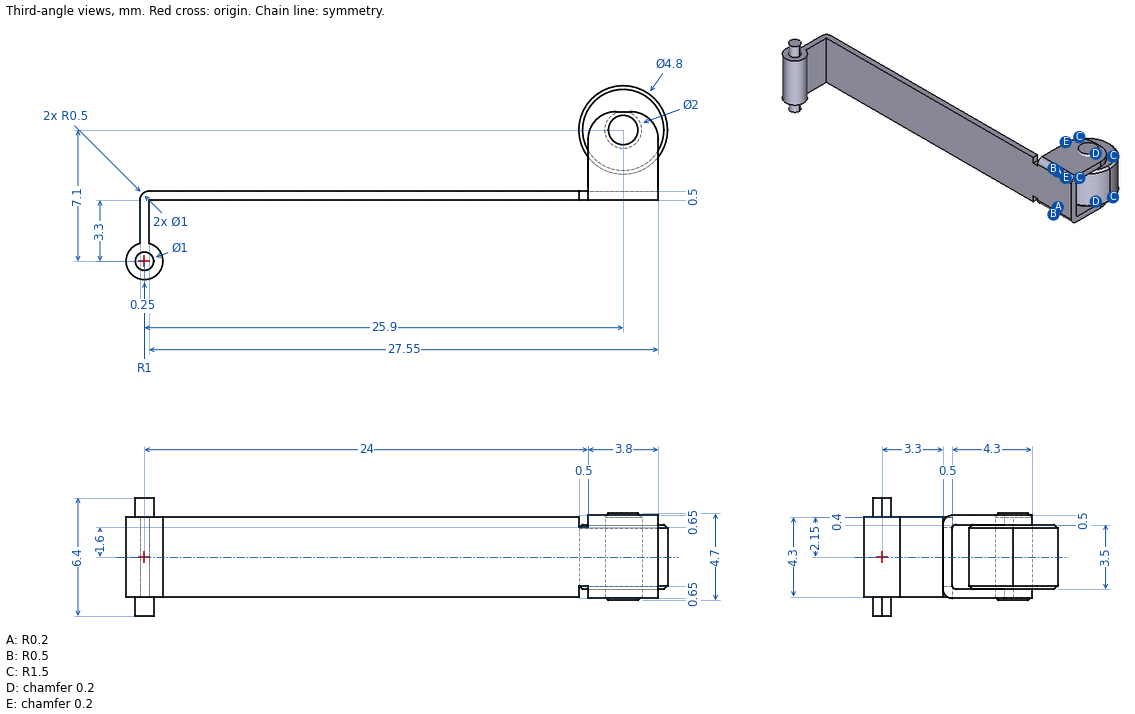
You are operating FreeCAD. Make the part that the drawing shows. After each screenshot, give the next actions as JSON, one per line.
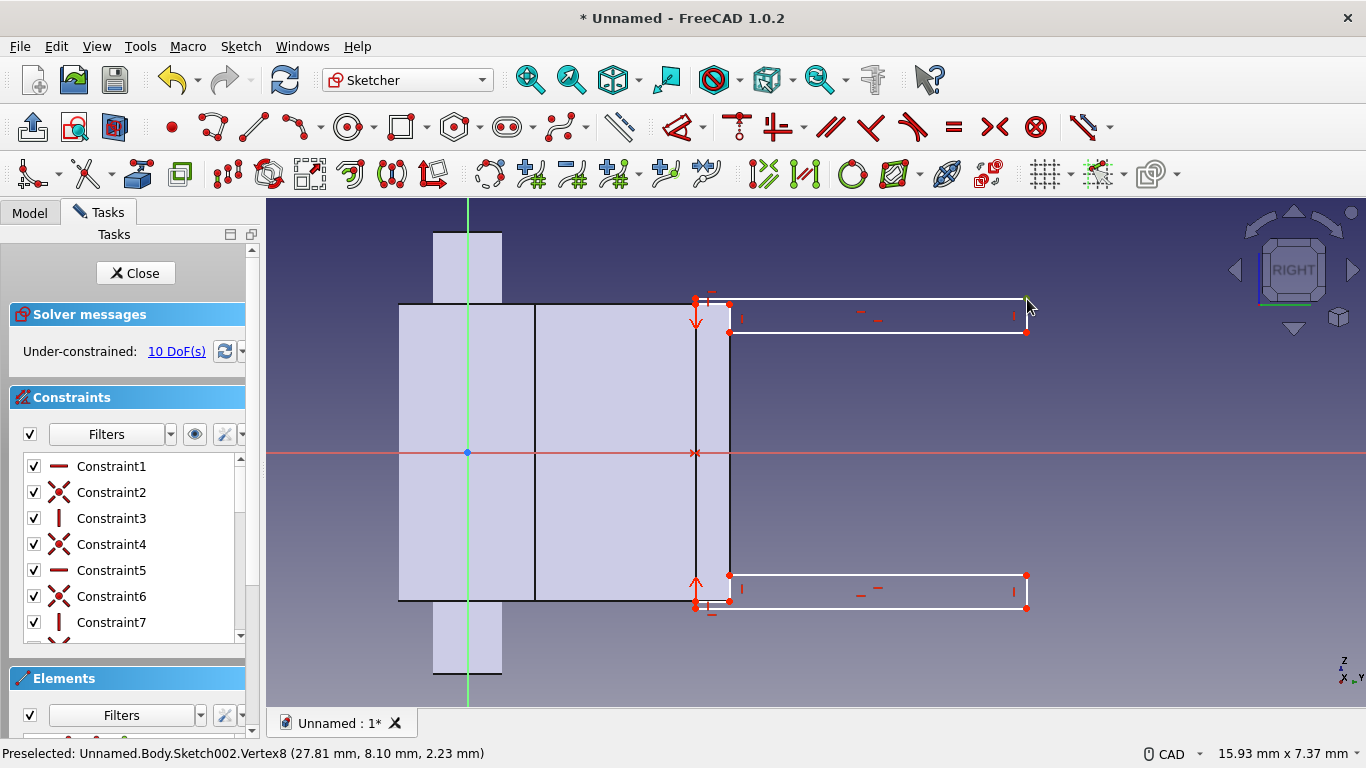
{"action": "left_click", "coordinate": [1027, 609]}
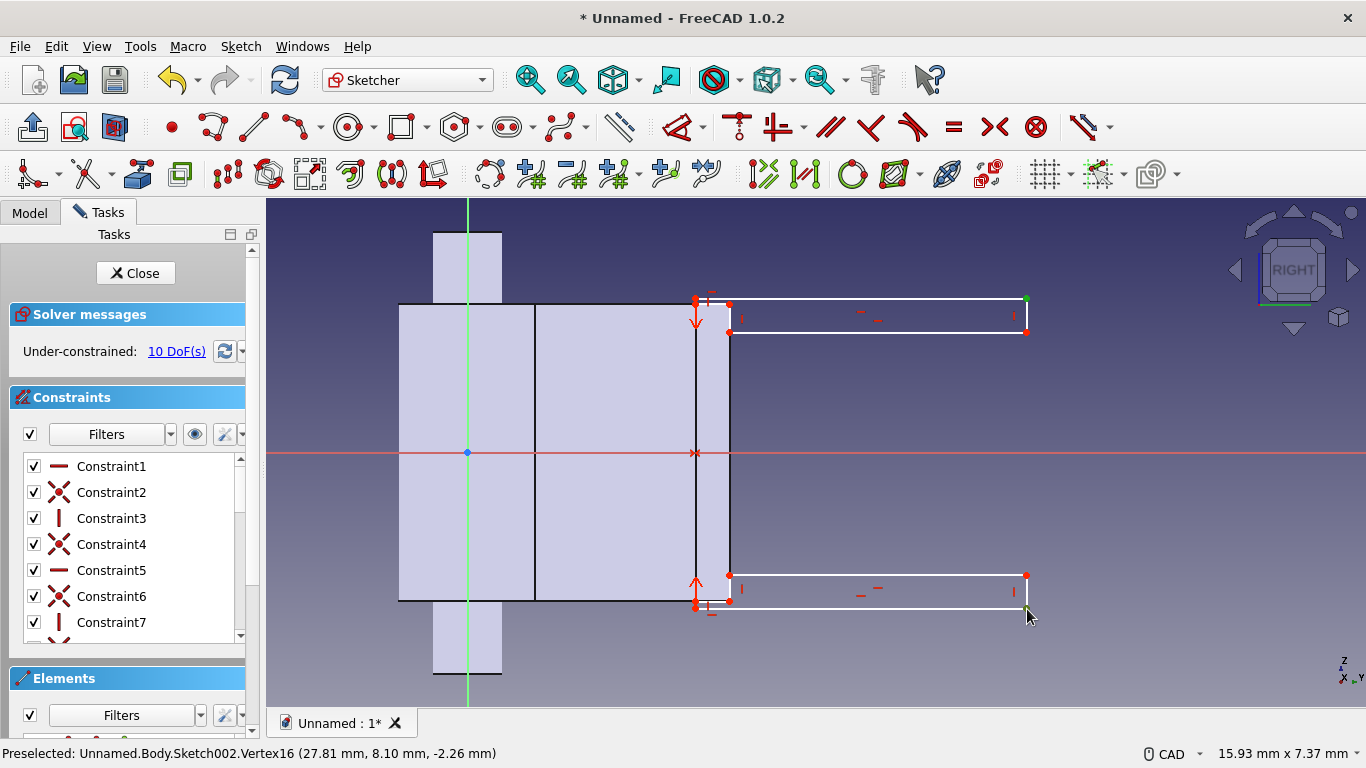
{"action": "left_click", "coordinate": [359, 453]}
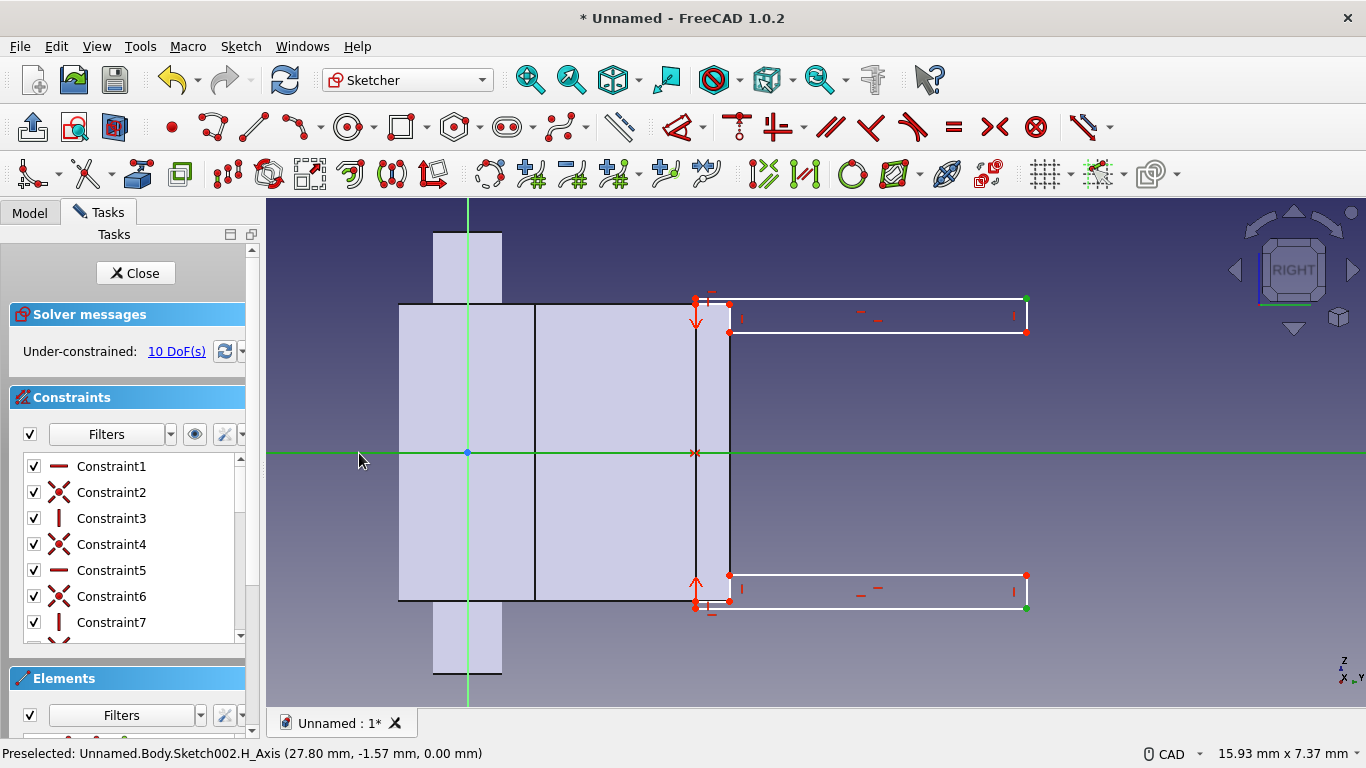
{"action": "key", "text": "s"}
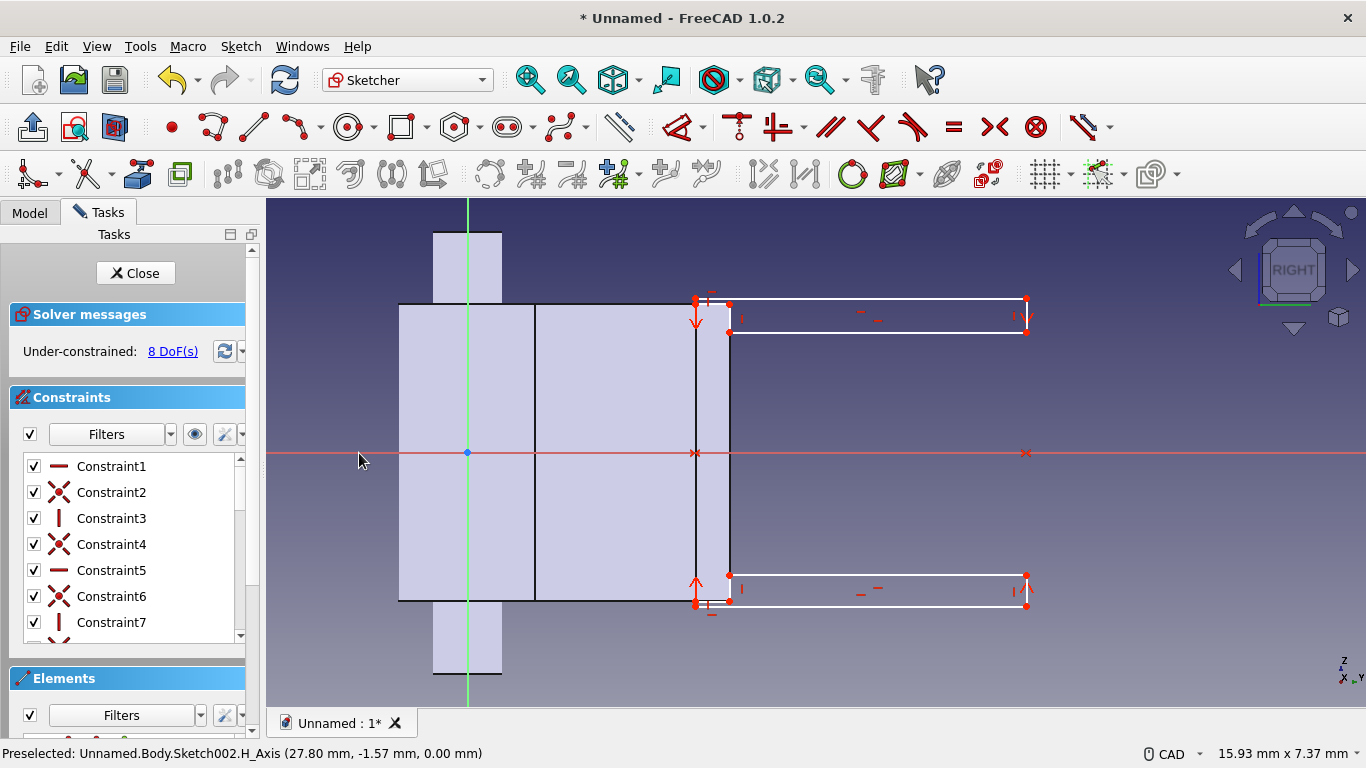
{"action": "left_click", "coordinate": [730, 333]}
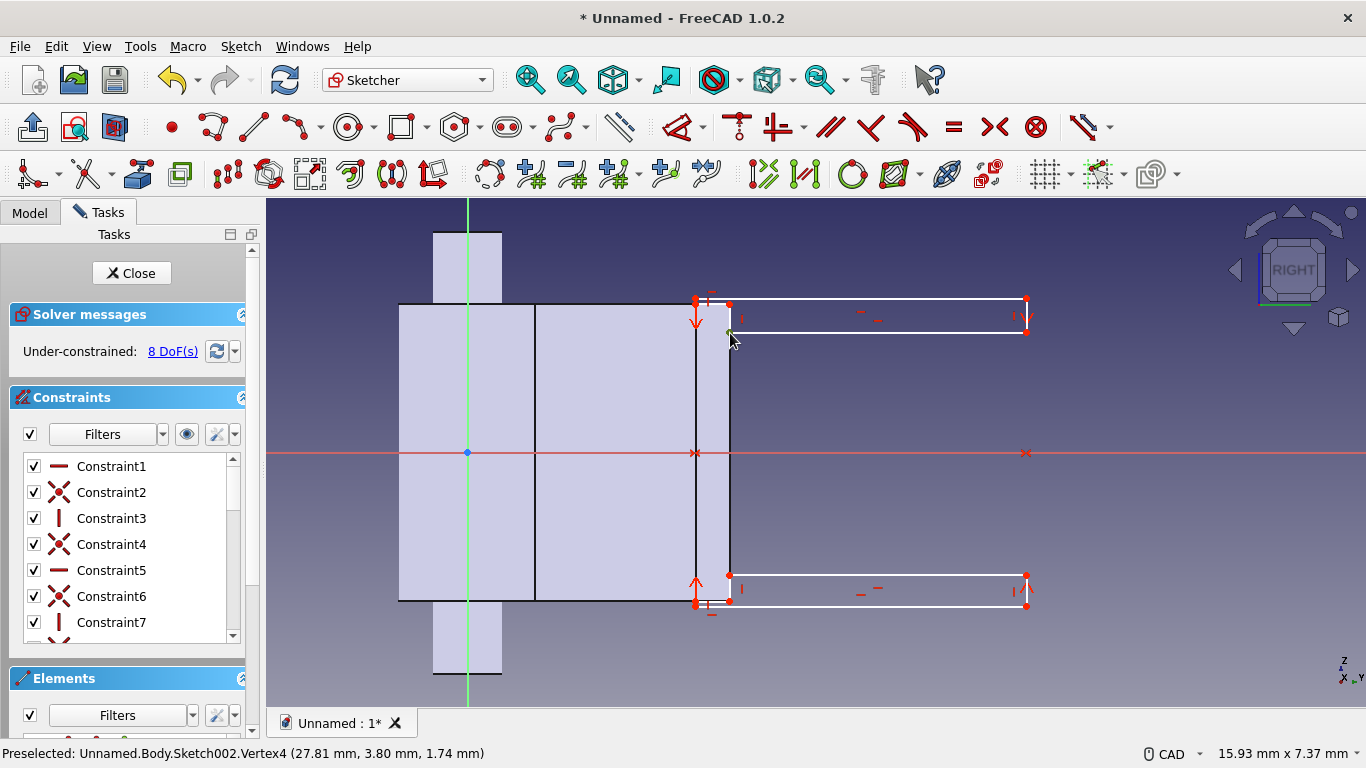
{"action": "left_click", "coordinate": [730, 575]}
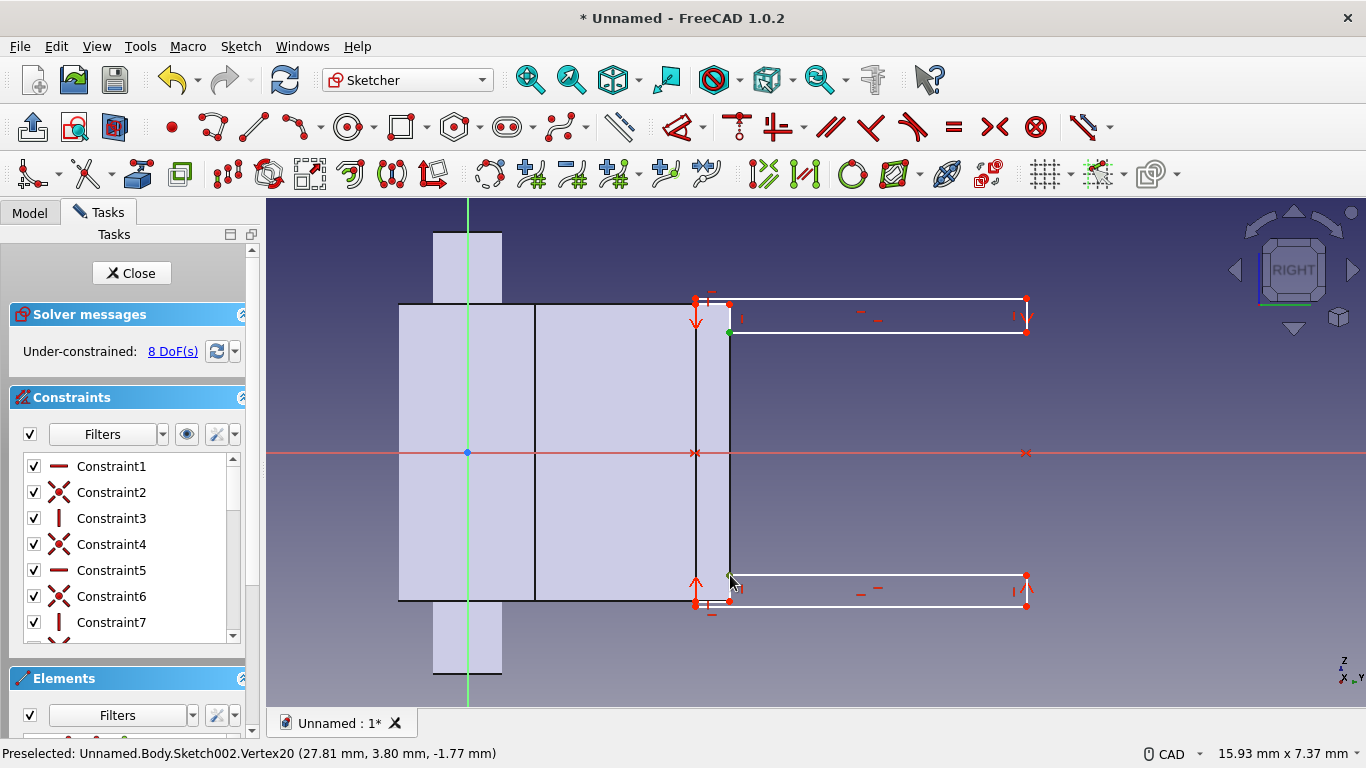
{"action": "left_click", "coordinate": [359, 453]}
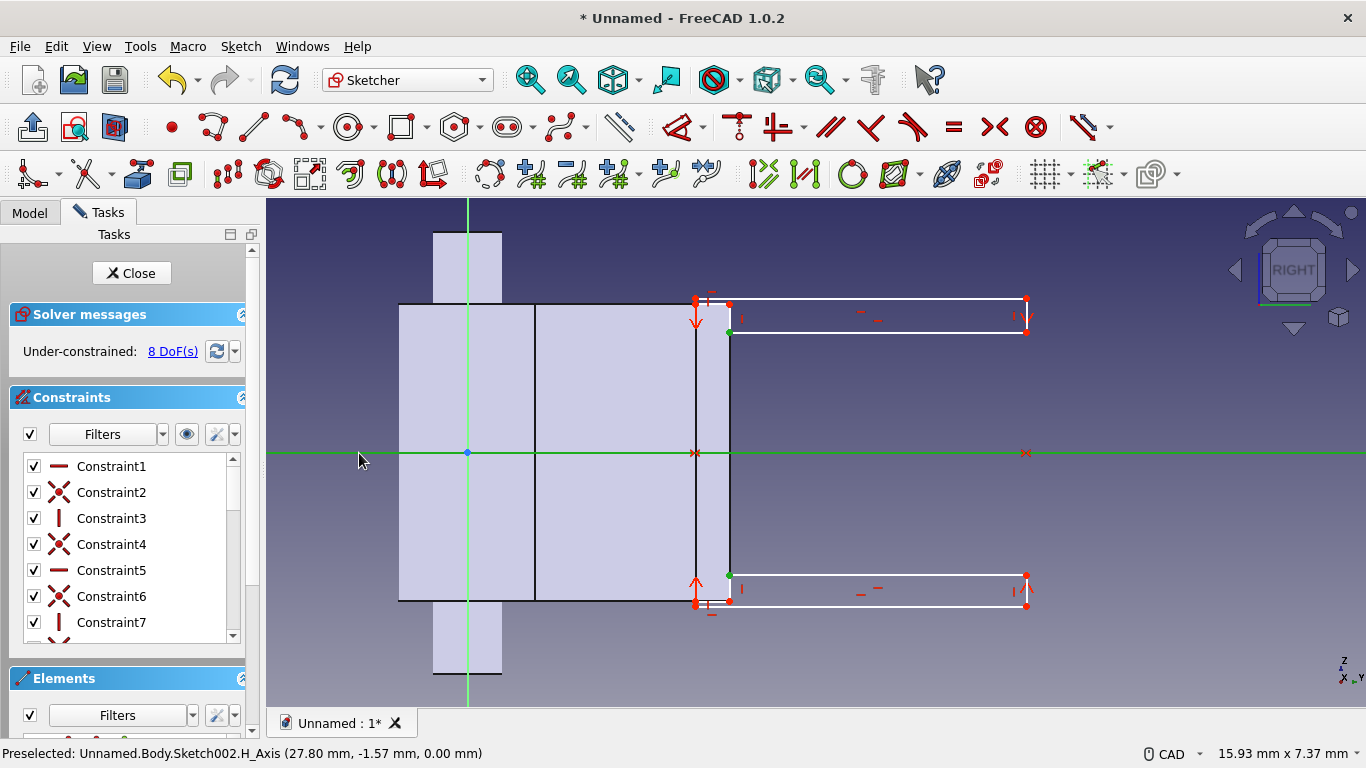
{"action": "left_click", "coordinate": [995, 128]}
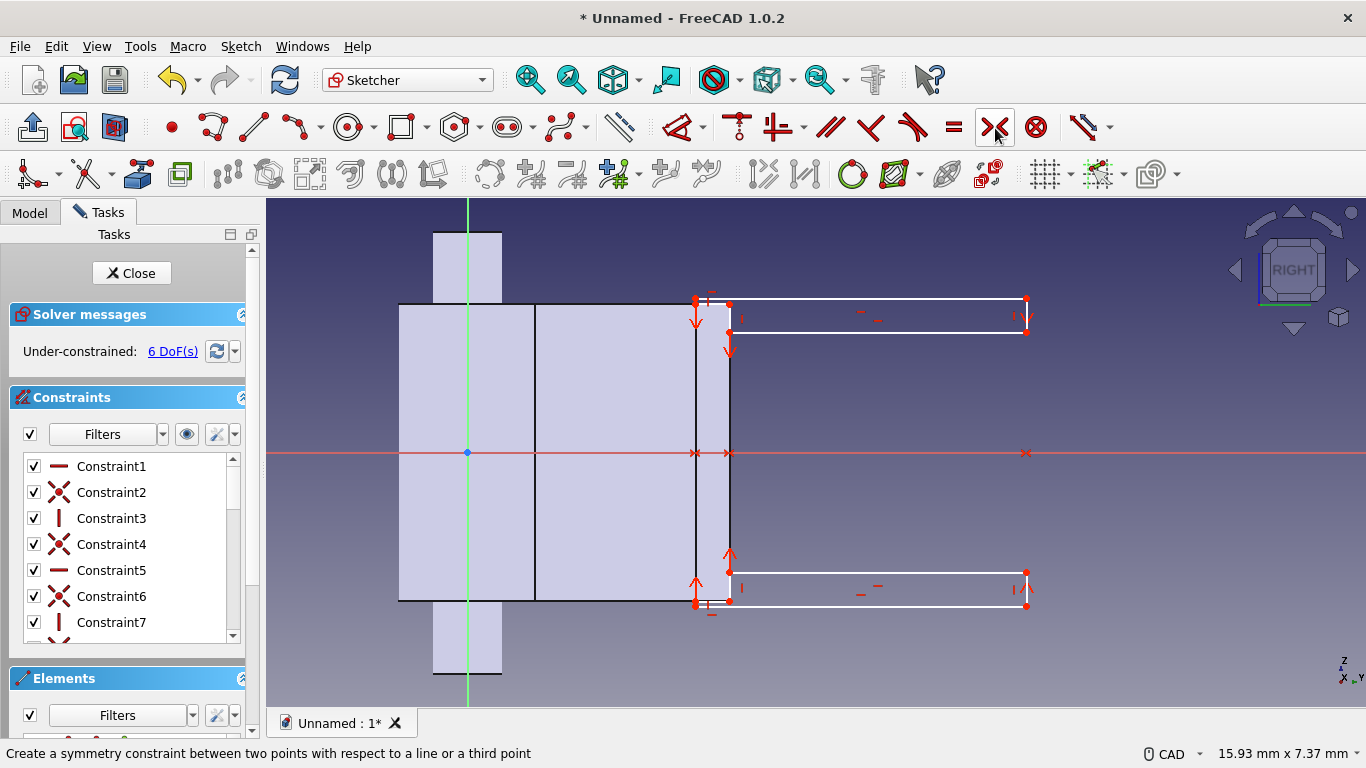
{"action": "key", "text": "d"}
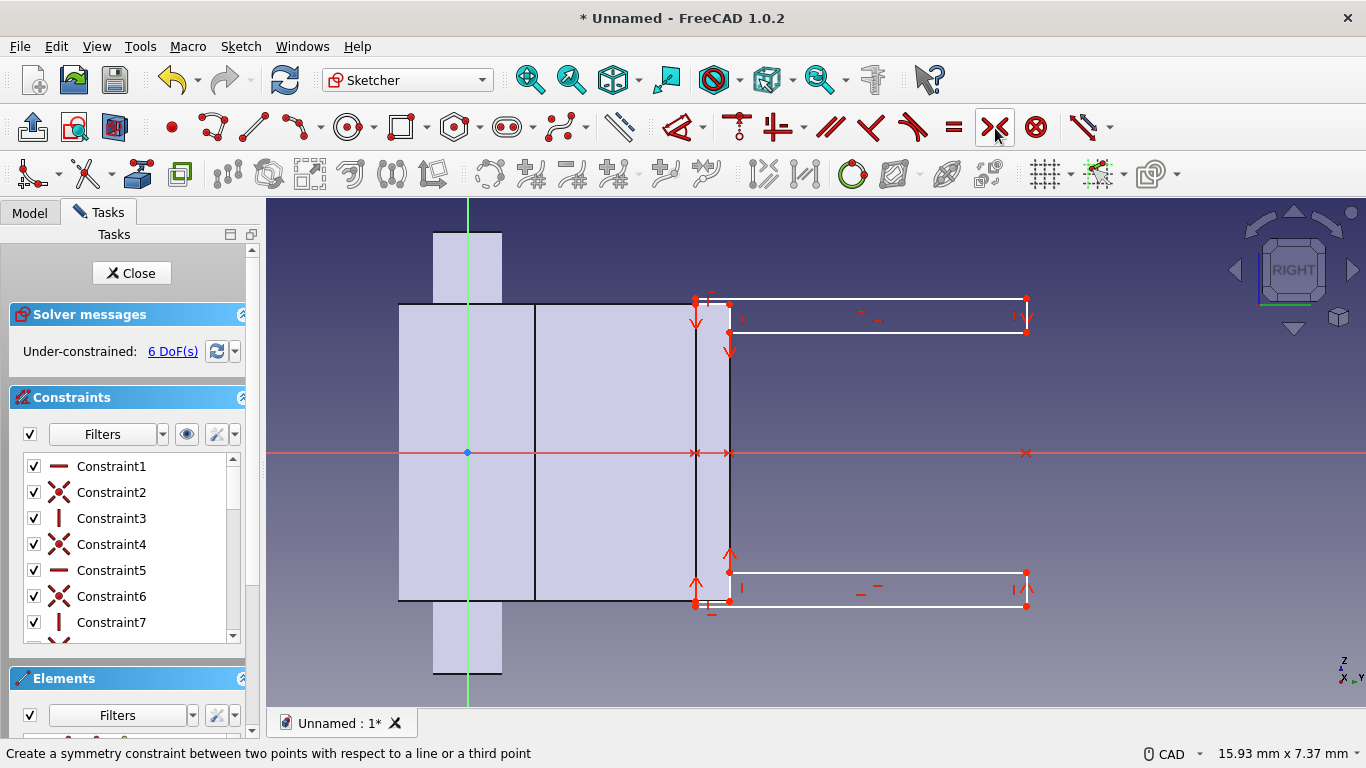
{"action": "scroll", "coordinate": [706, 304], "scroll_direction": "up", "scroll_amount": 5}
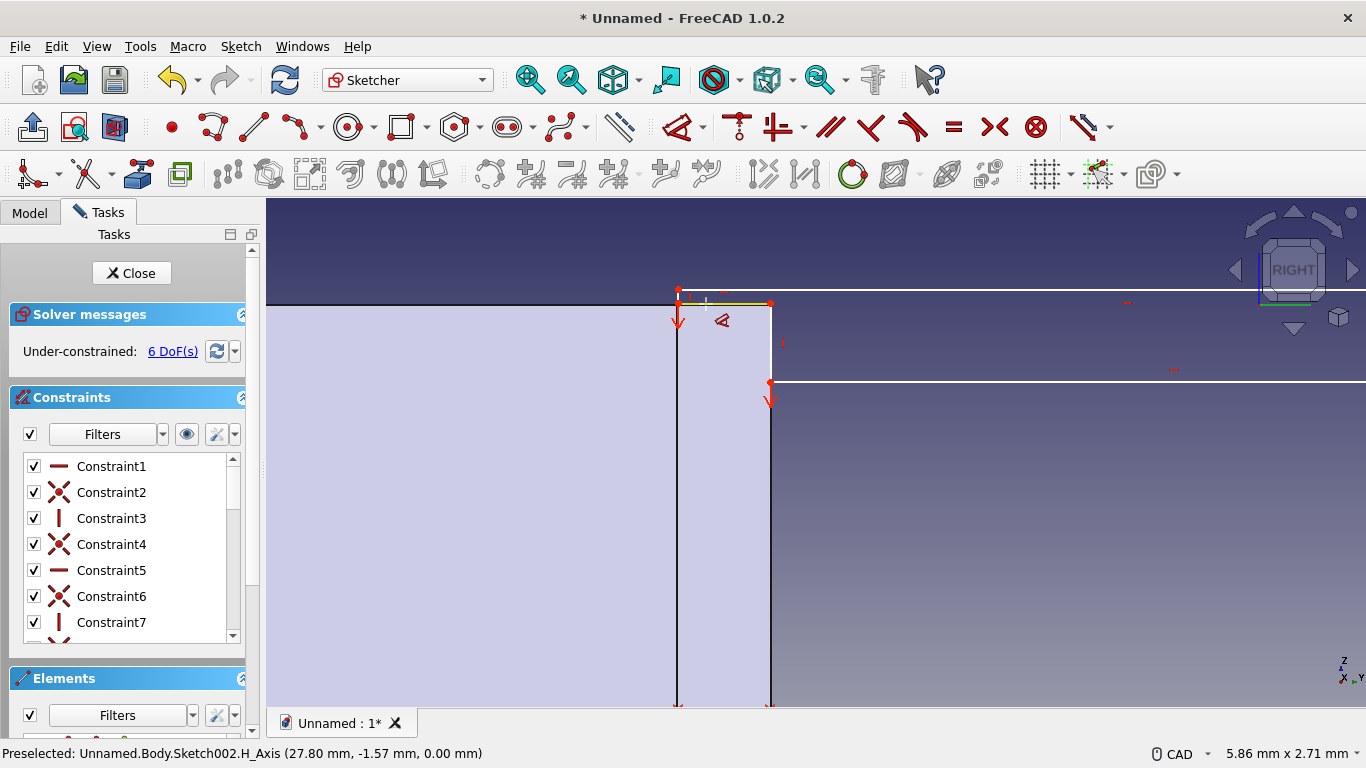
{"action": "left_click", "coordinate": [706, 304]}
{"action": "left_click", "coordinate": [724, 270]}